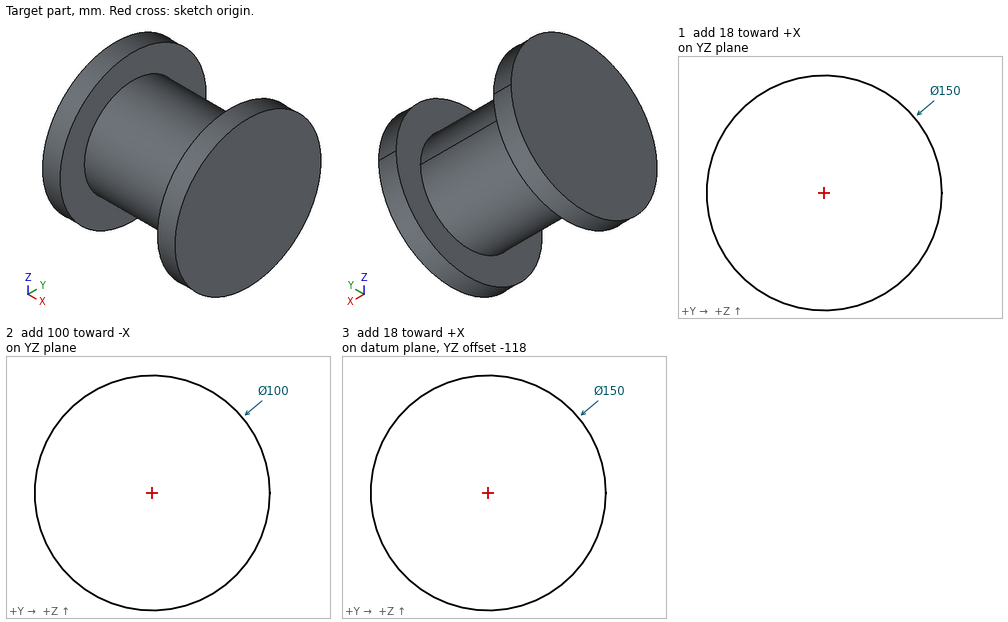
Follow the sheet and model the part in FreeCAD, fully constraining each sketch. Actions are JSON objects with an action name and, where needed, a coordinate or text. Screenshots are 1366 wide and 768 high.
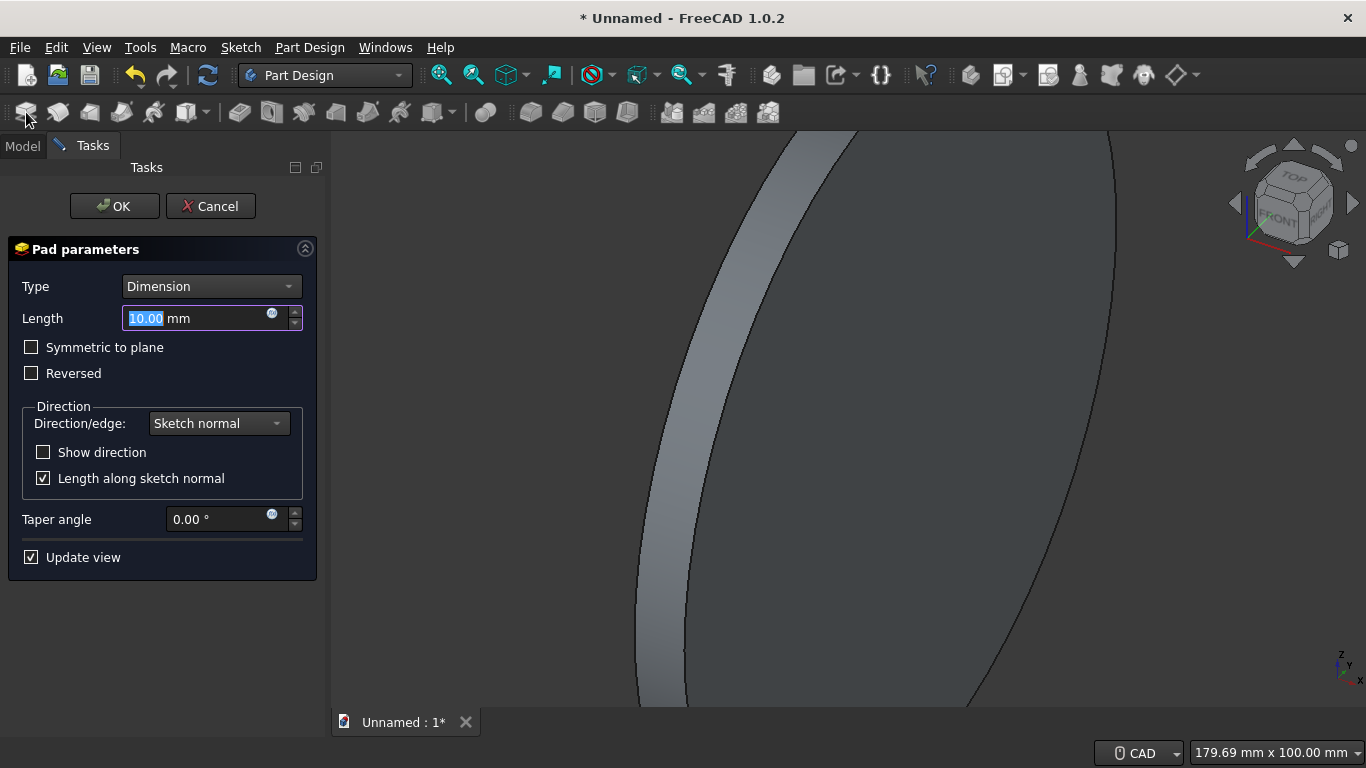
{"action": "type", "text": "18"}
{"action": "key", "text": "Tab"}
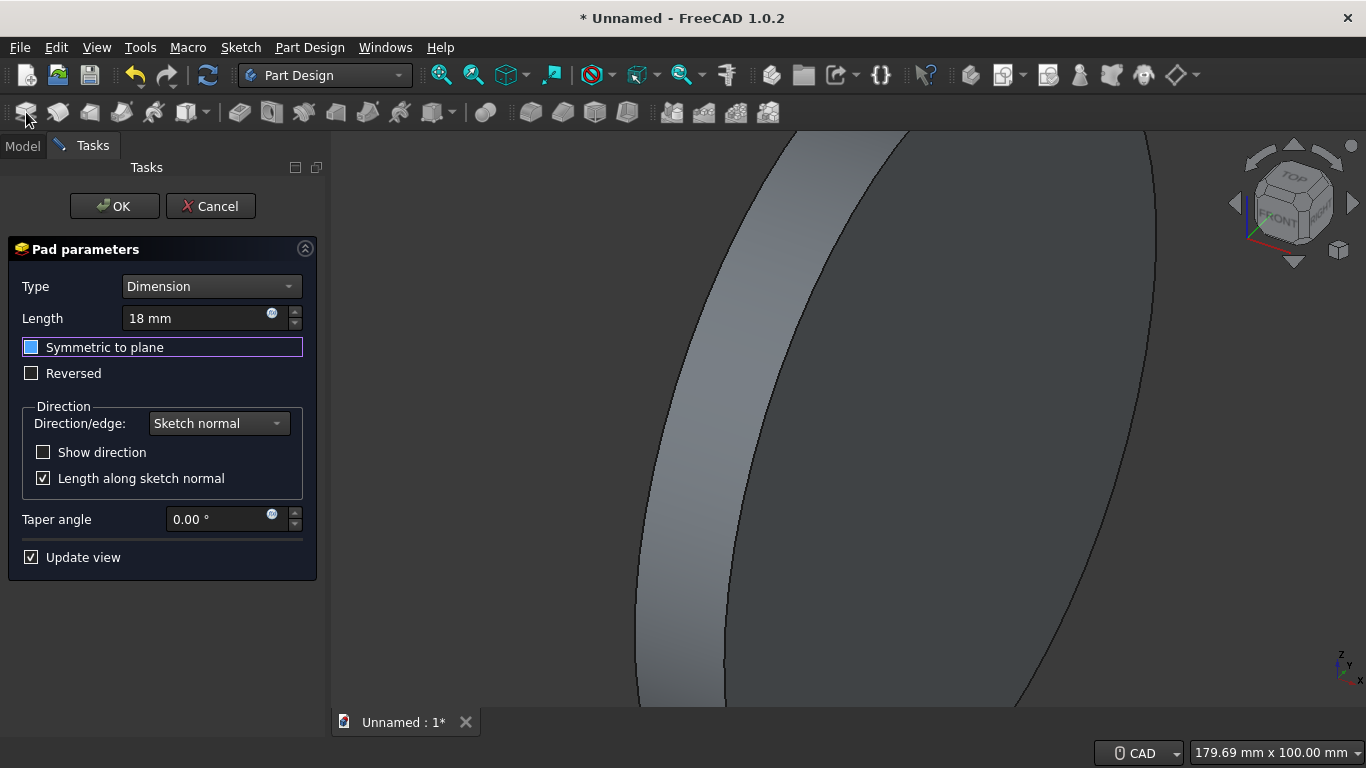
{"action": "left_click", "coordinate": [115, 206]}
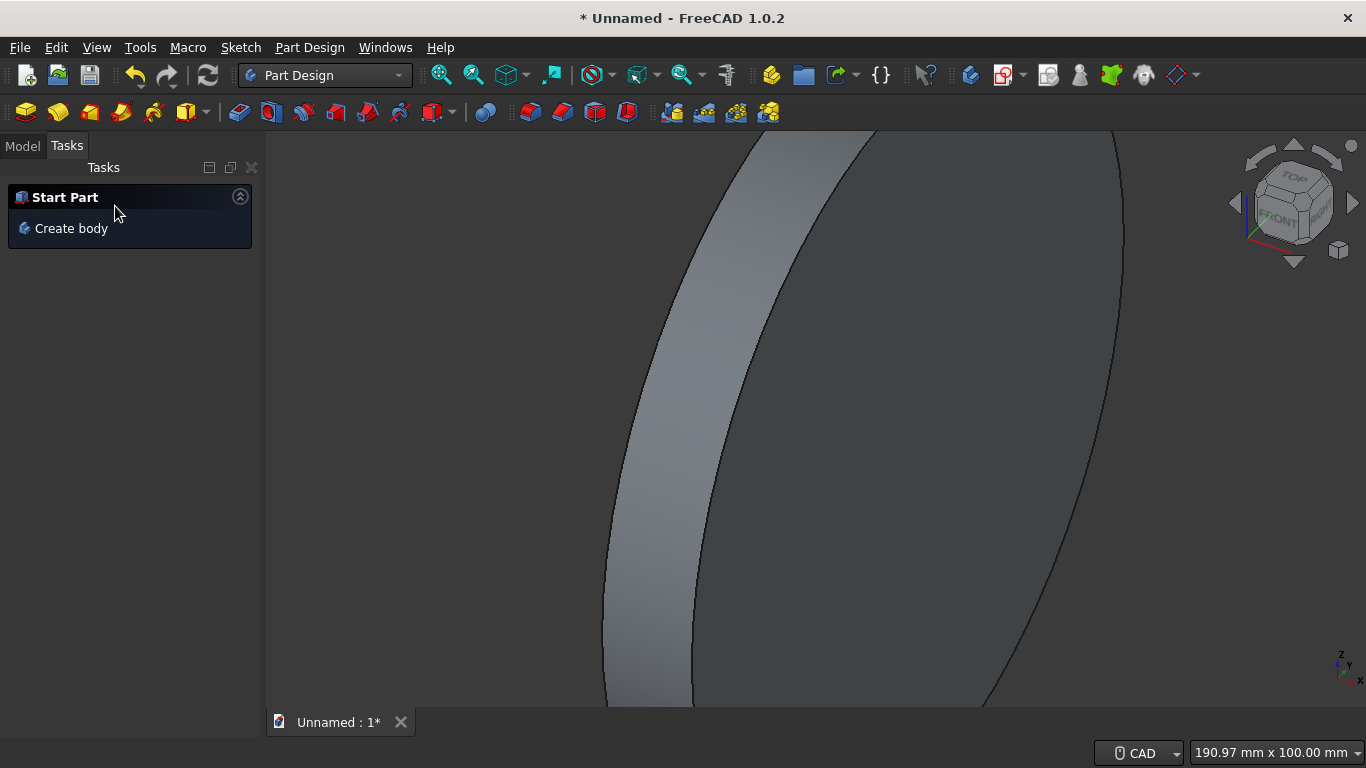
{"action": "left_click", "coordinate": [442, 76]}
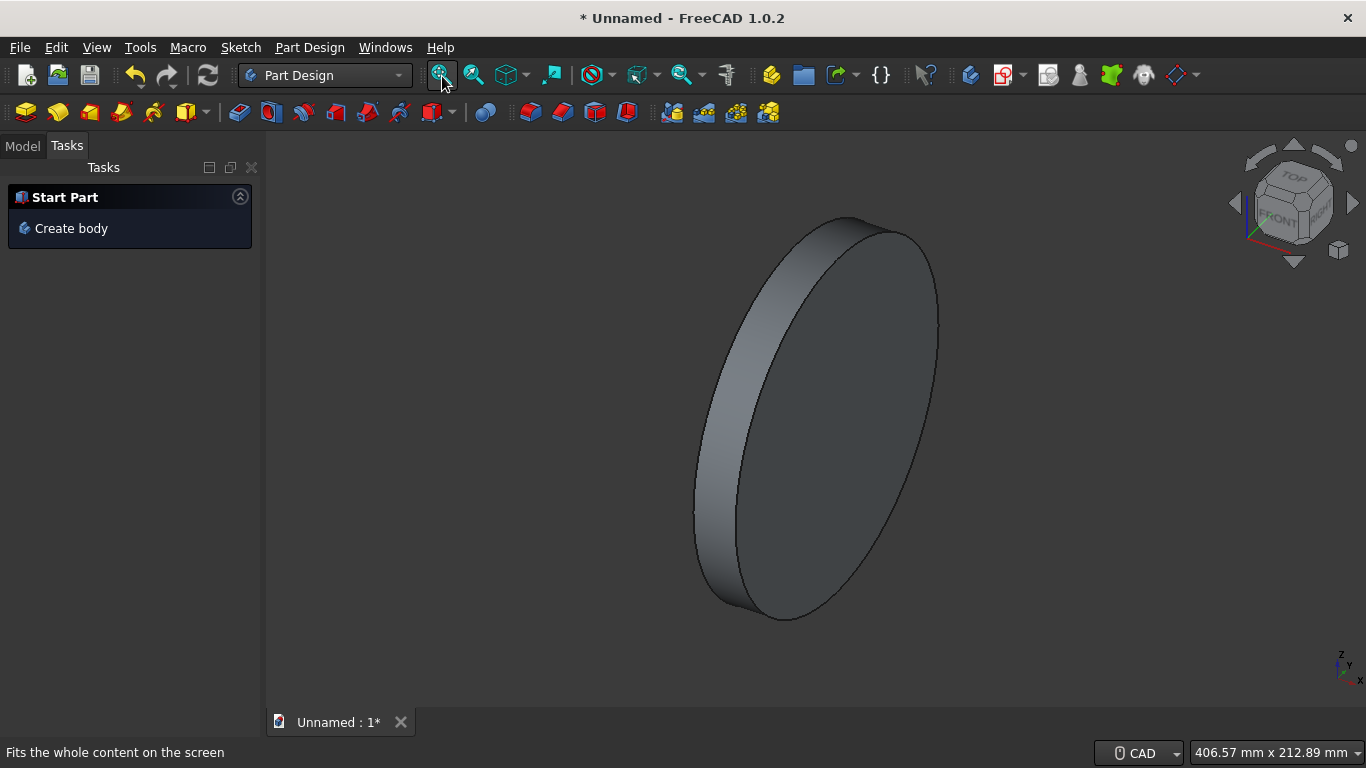
{"action": "left_click", "coordinate": [1004, 76]}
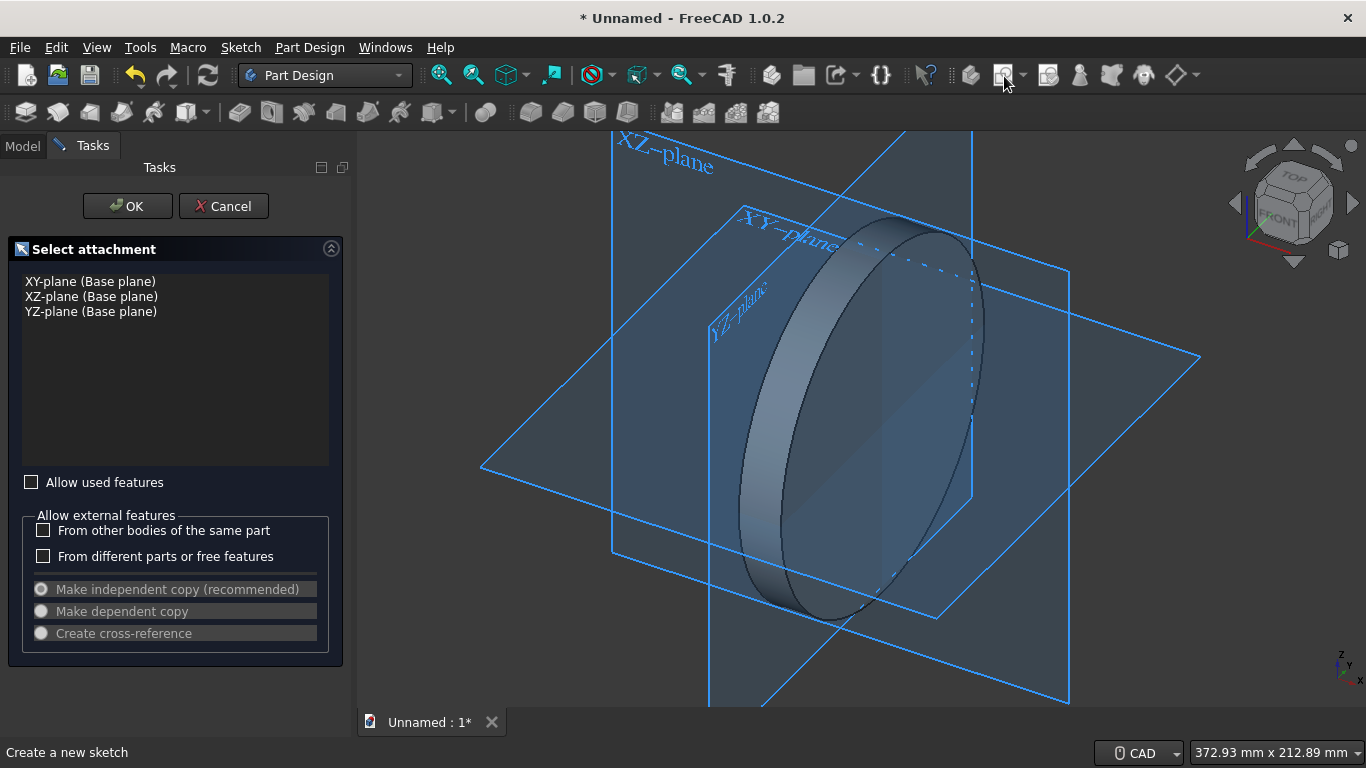
{"action": "left_click", "coordinate": [82, 312]}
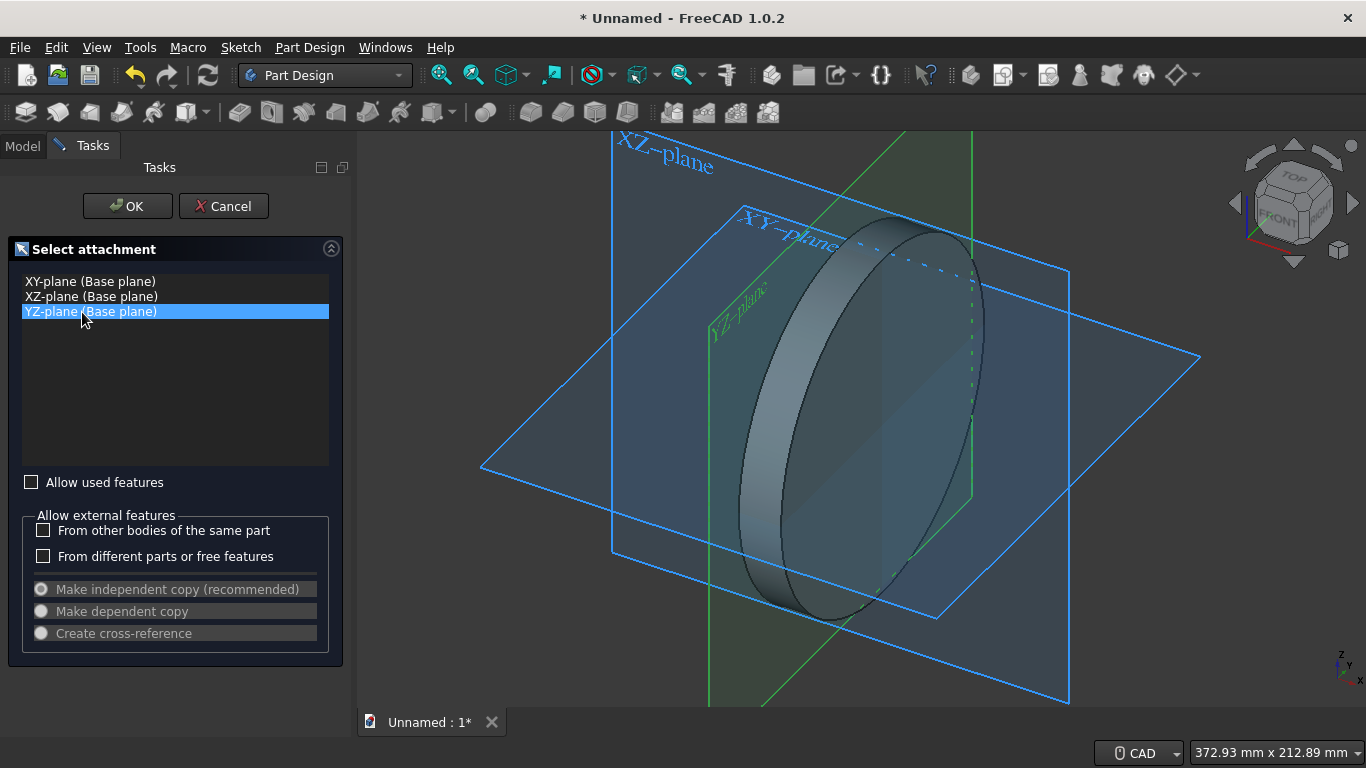
{"action": "left_click", "coordinate": [128, 206]}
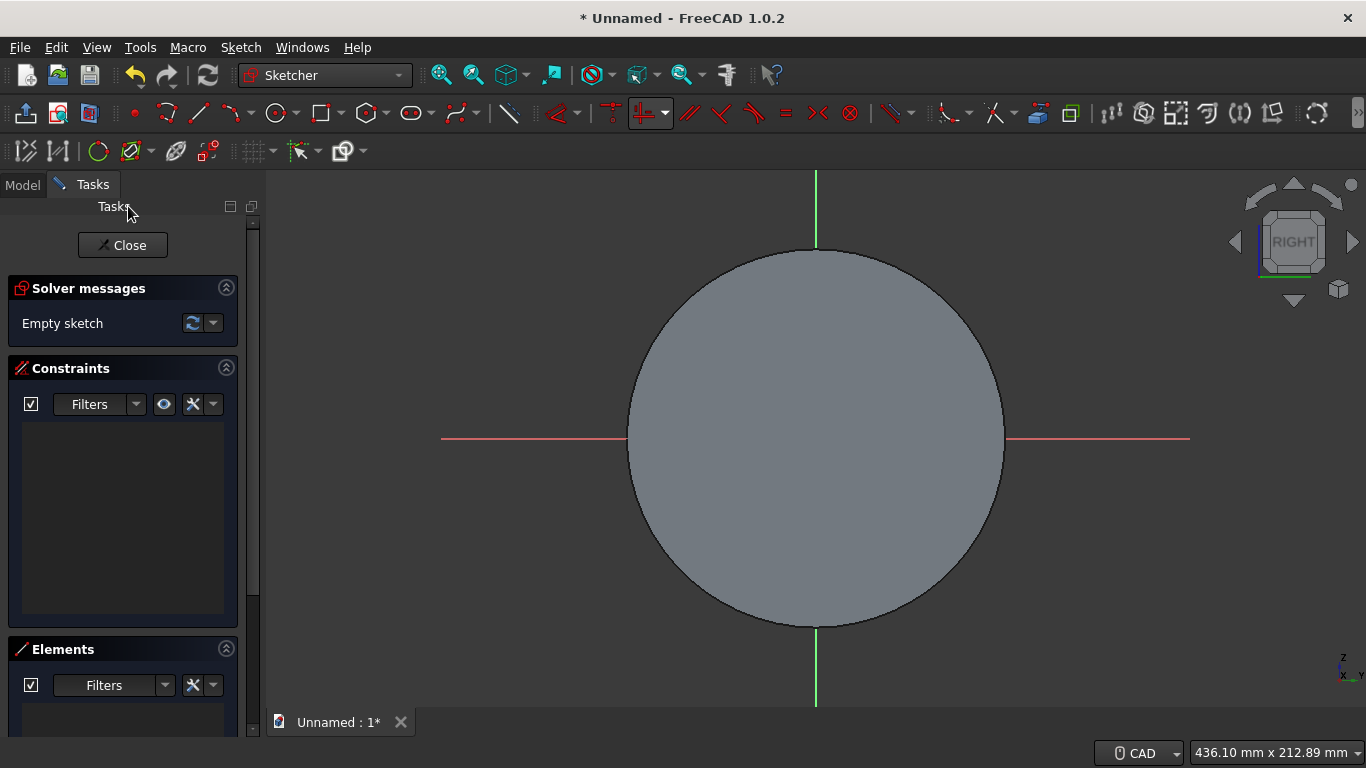
{"action": "left_click", "coordinate": [90, 114]}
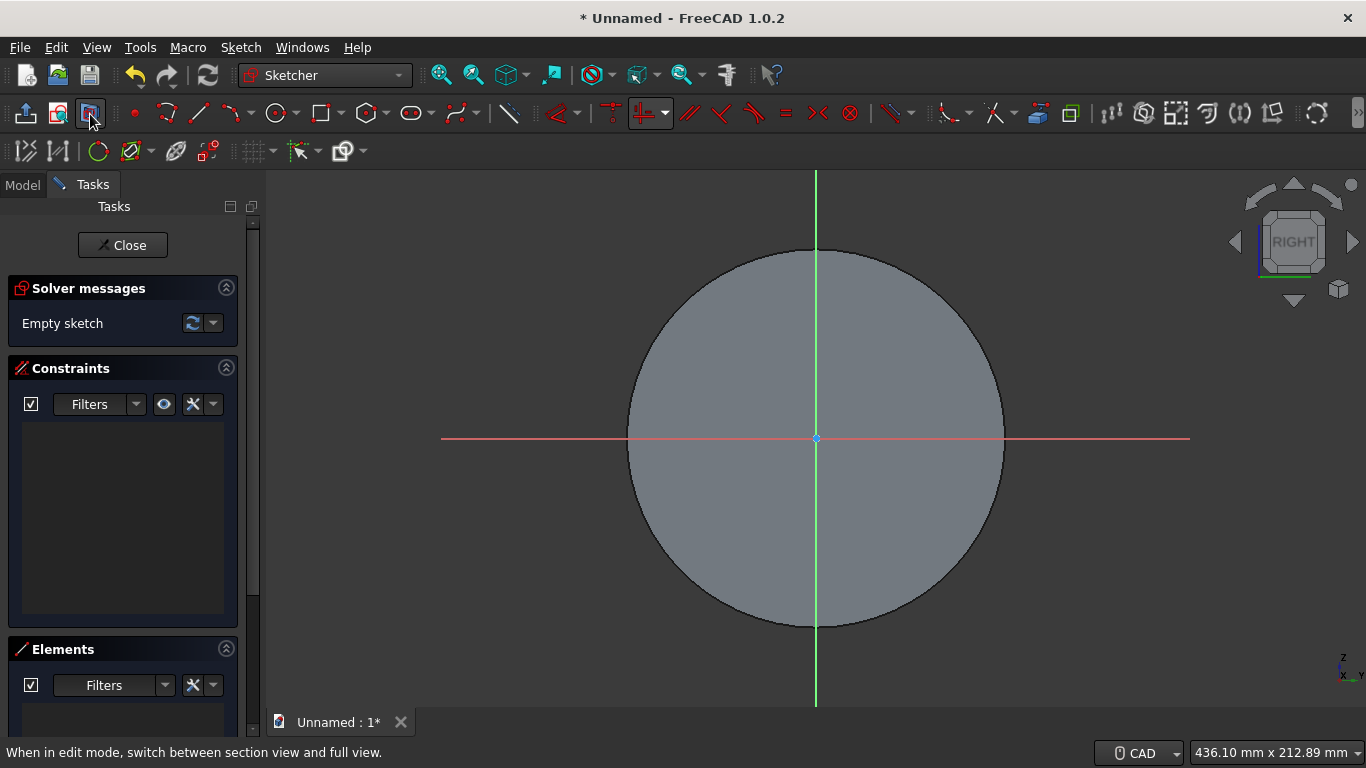
{"action": "left_click", "coordinate": [276, 114]}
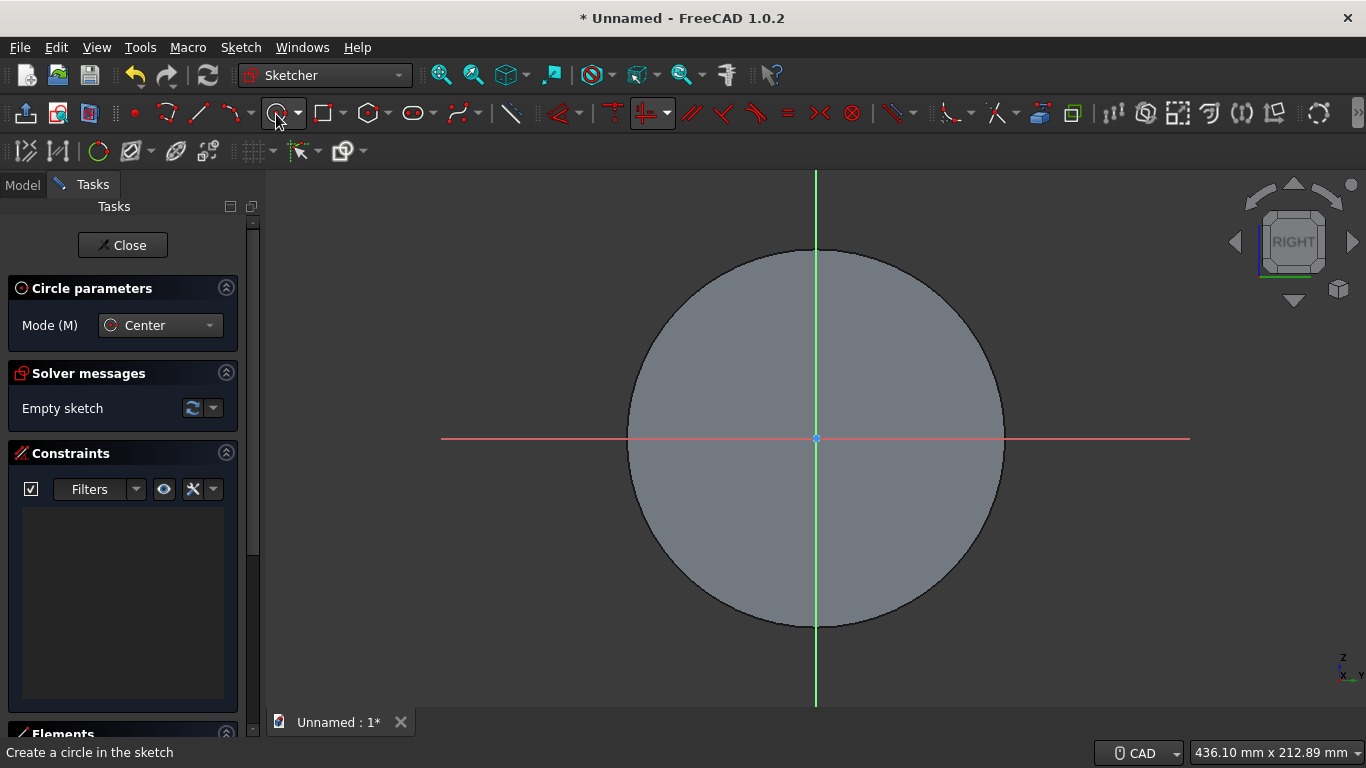
{"action": "left_click", "coordinate": [816, 438]}
{"action": "mouse_move", "coordinate": [905, 349]}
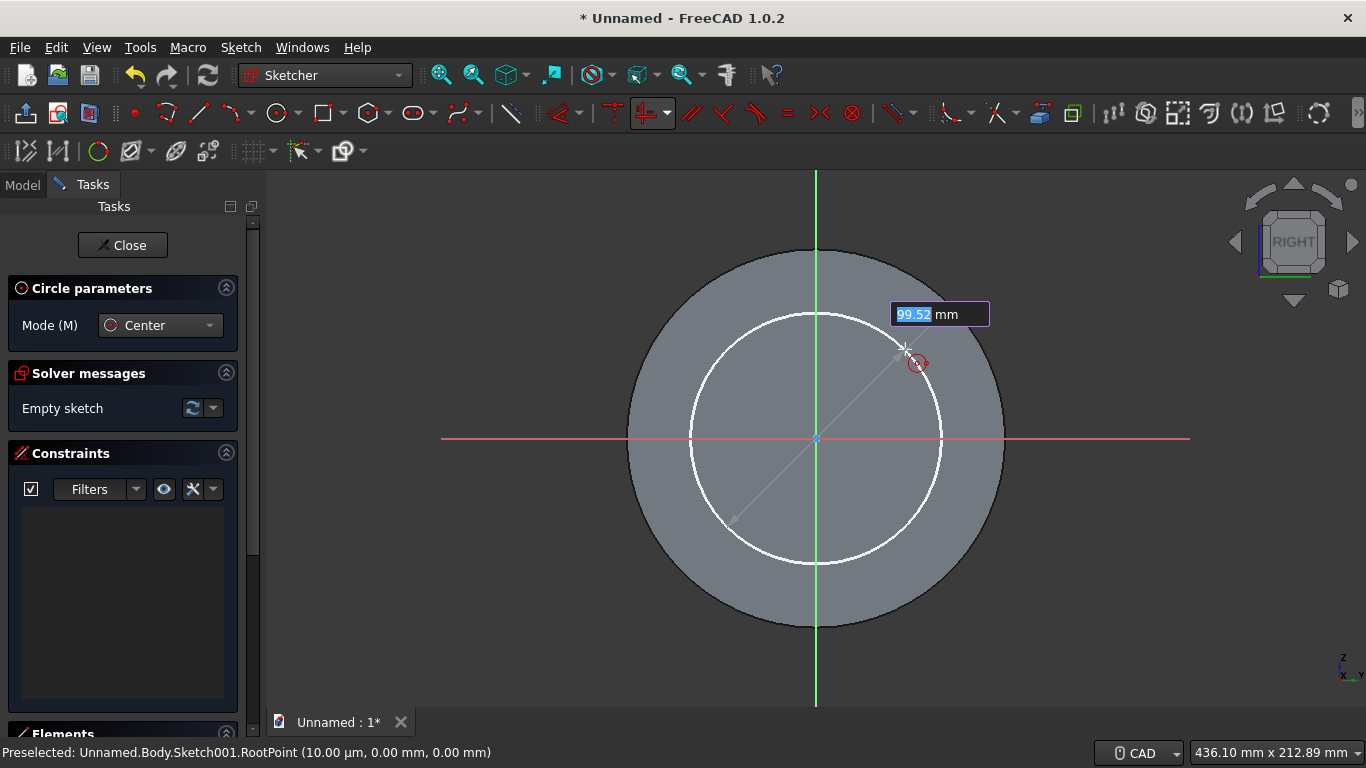
{"action": "type", "text": "100"}
{"action": "key", "text": "Return"}
{"action": "key", "text": "Escape"}